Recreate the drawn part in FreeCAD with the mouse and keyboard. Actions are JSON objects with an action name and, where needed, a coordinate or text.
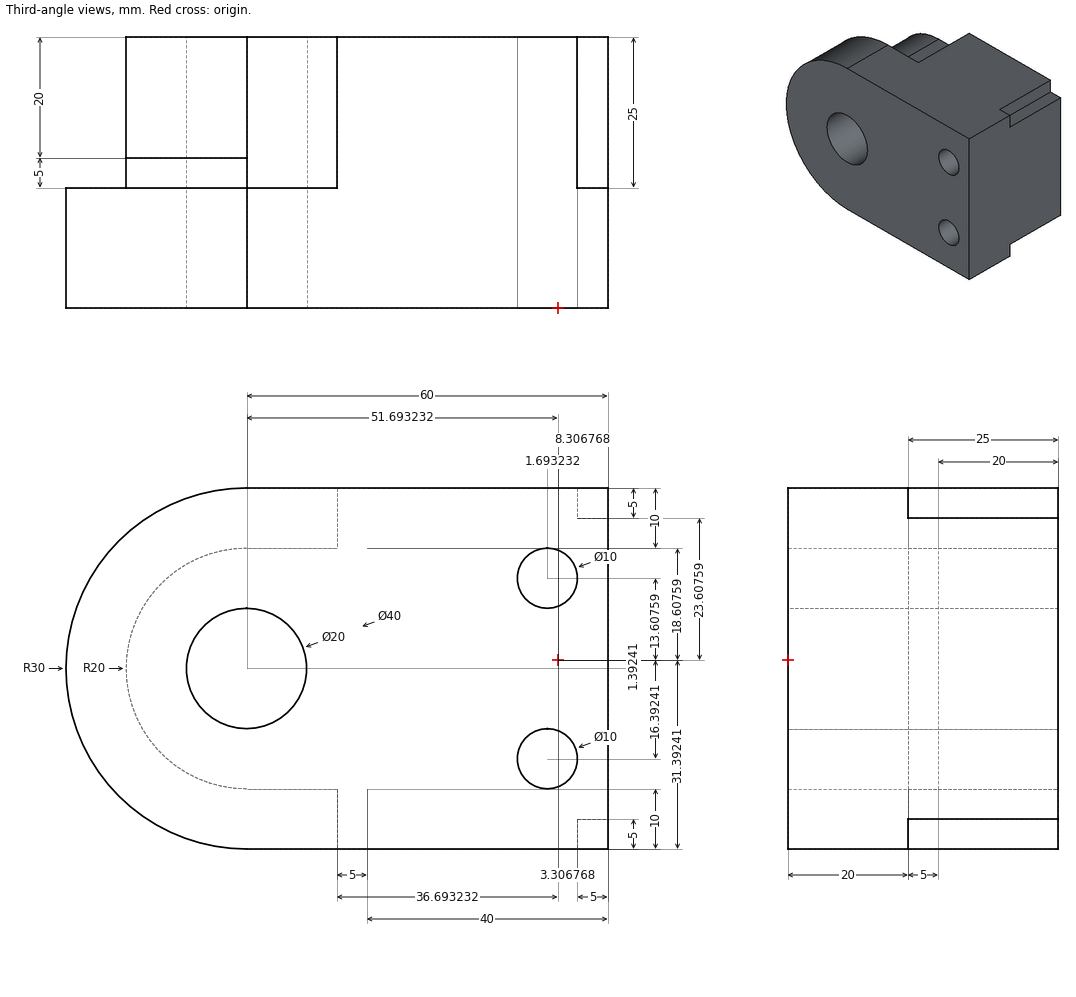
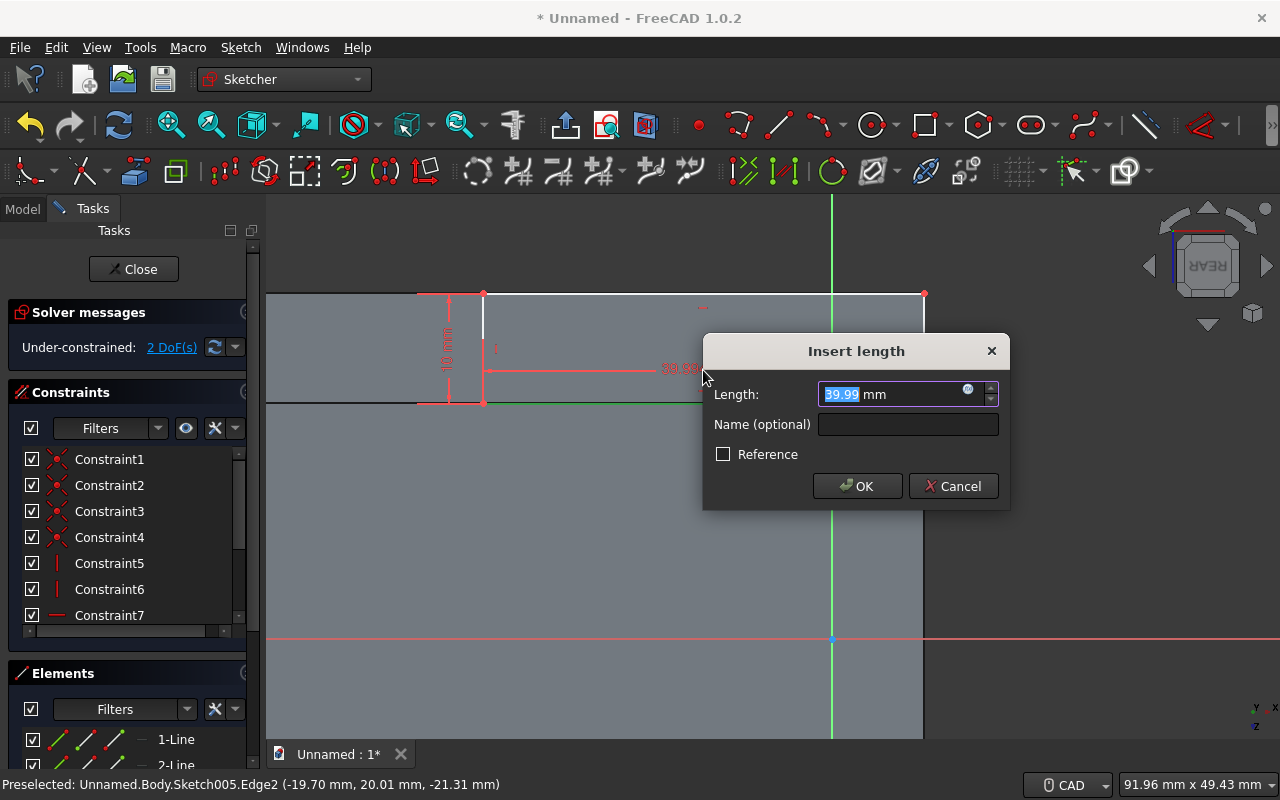
{"action": "type", "text": "40"}
{"action": "key", "text": "Return"}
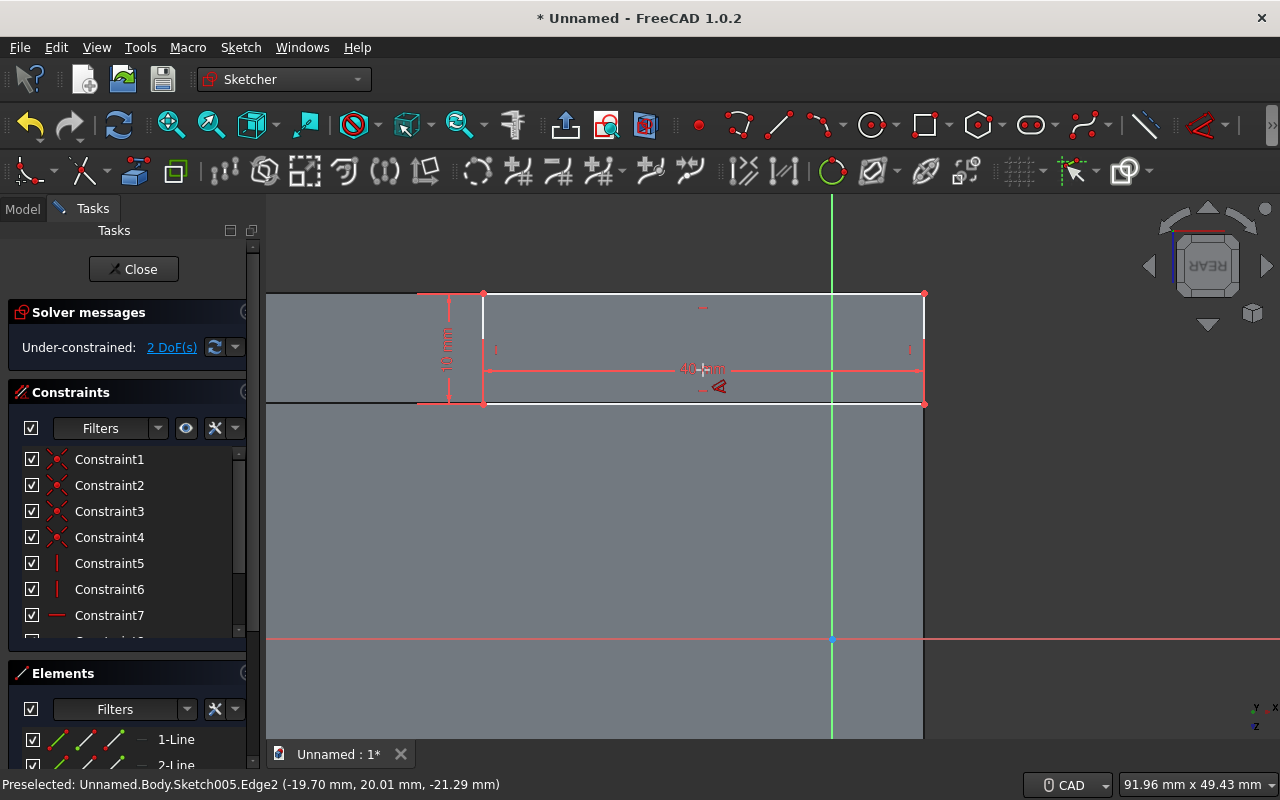
{"action": "left_click", "coordinate": [483, 294]}
{"action": "left_click", "coordinate": [449, 467]}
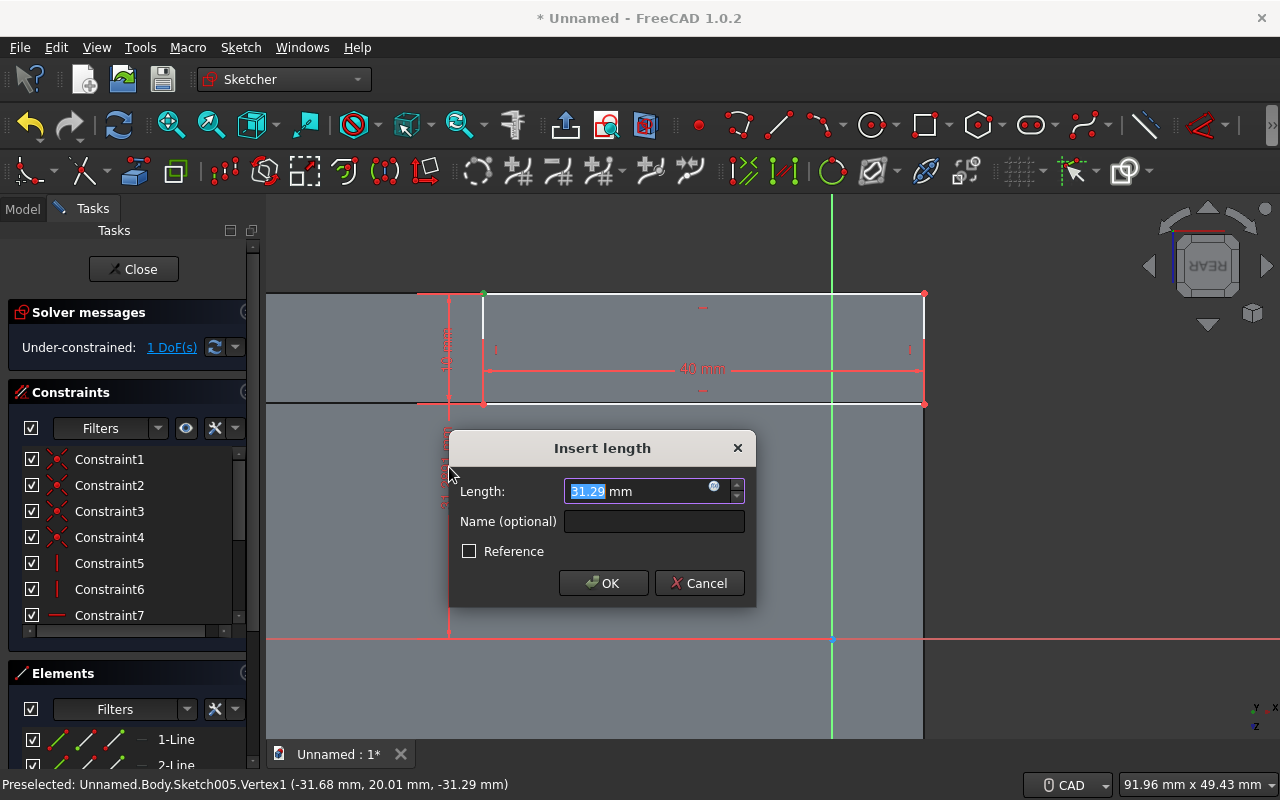
{"action": "type", "text": "31.39241"}
{"action": "key", "text": "Return"}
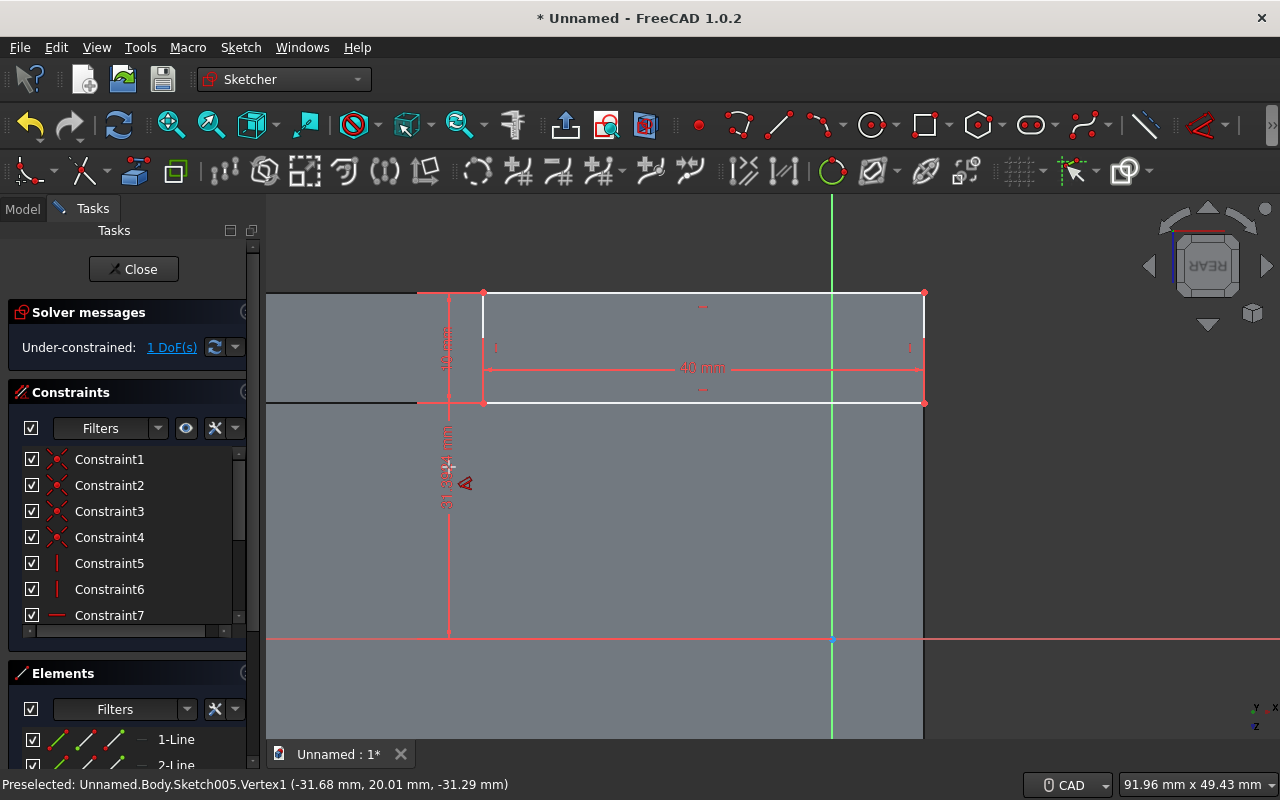
{"action": "left_click", "coordinate": [924, 403]}
{"action": "left_click", "coordinate": [878, 673]}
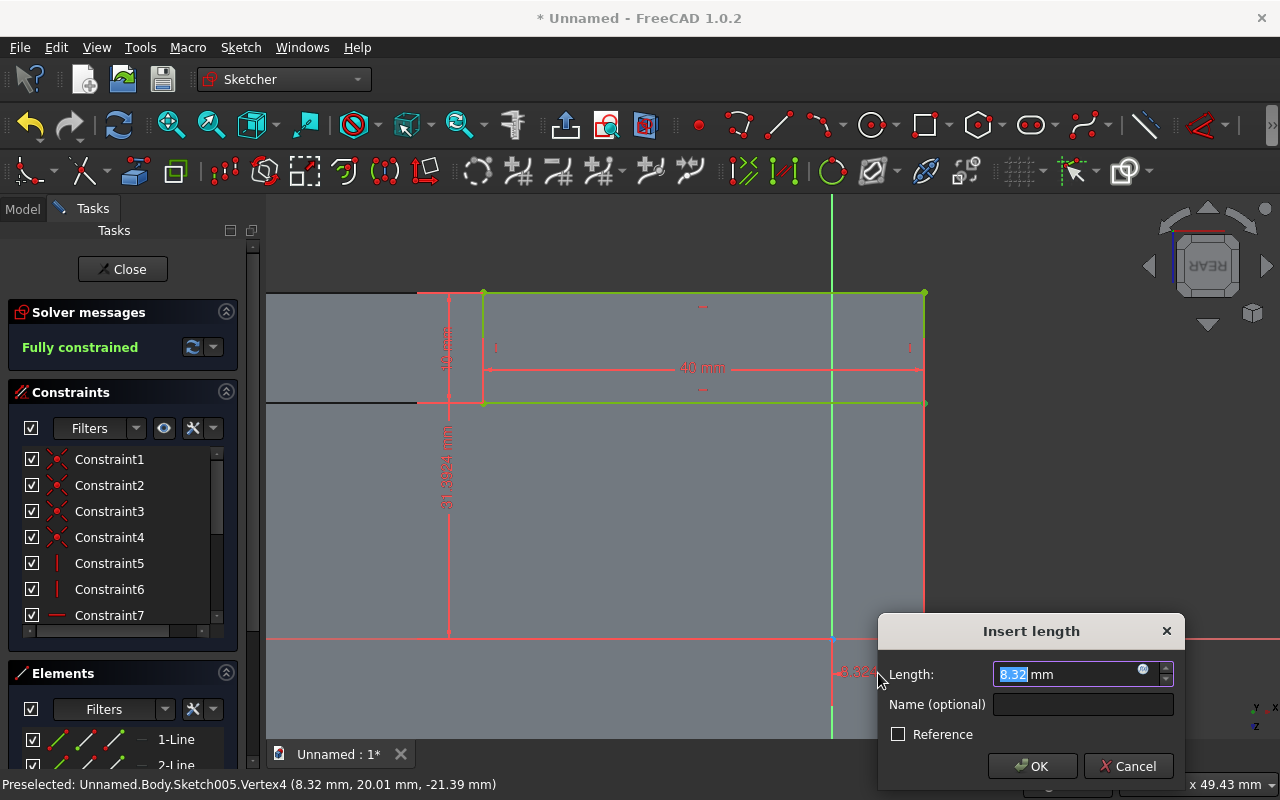
{"action": "type", "text": "8.306768"}
{"action": "key", "text": "Return"}
{"action": "key", "text": "Escape"}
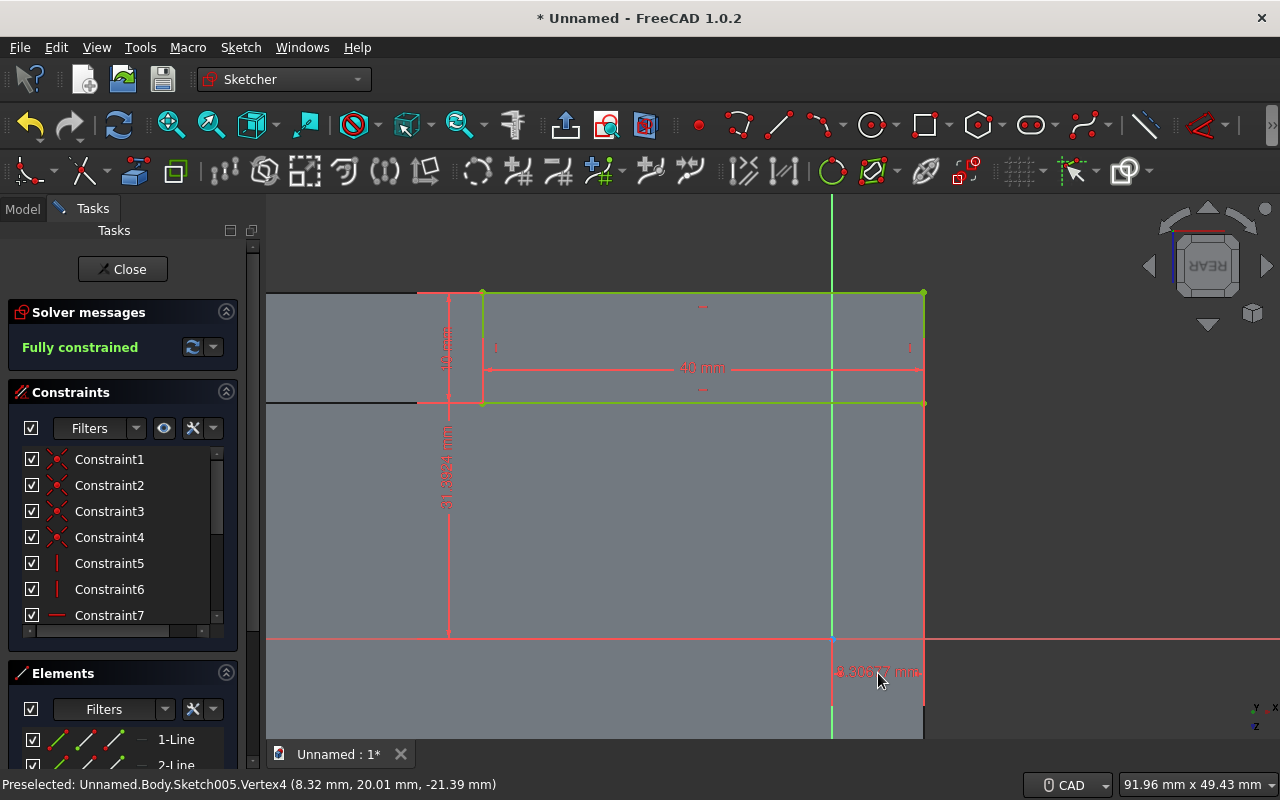
{"action": "left_click", "coordinate": [123, 269]}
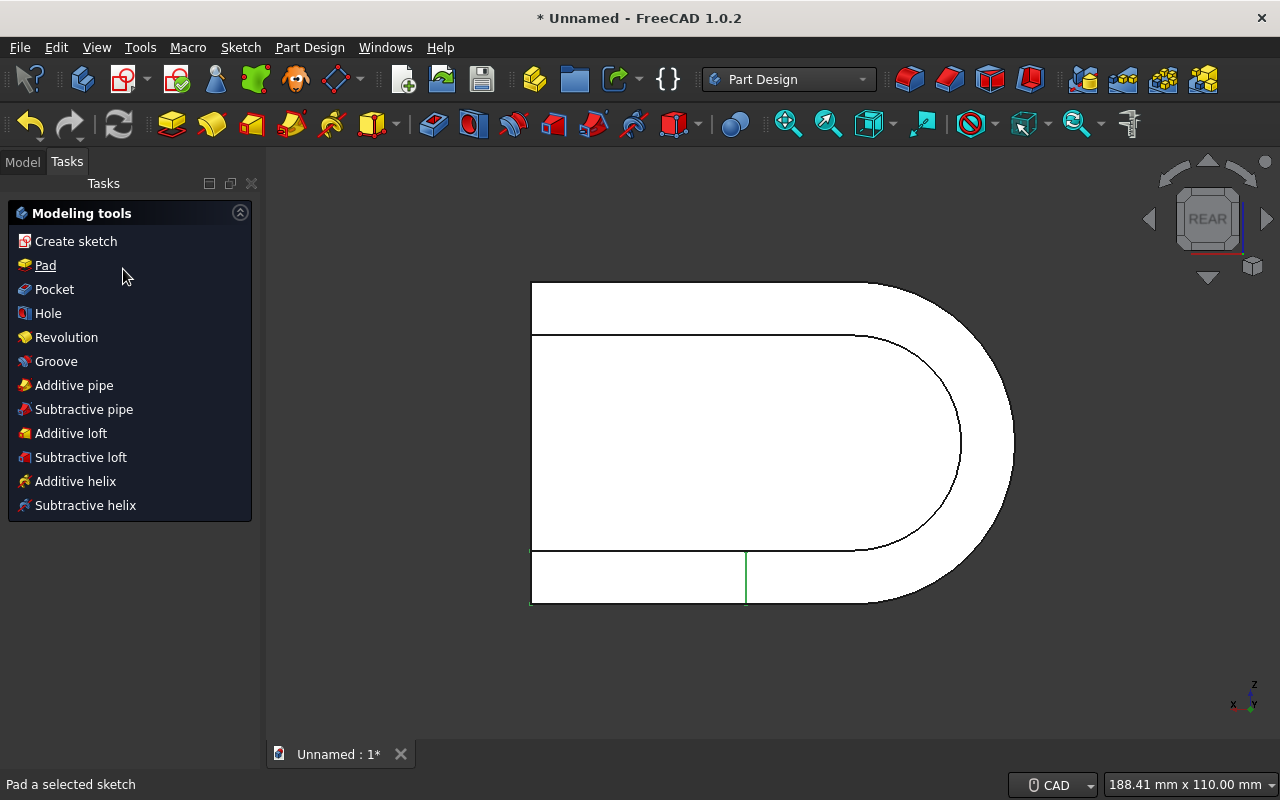
{"action": "left_click", "coordinate": [172, 124]}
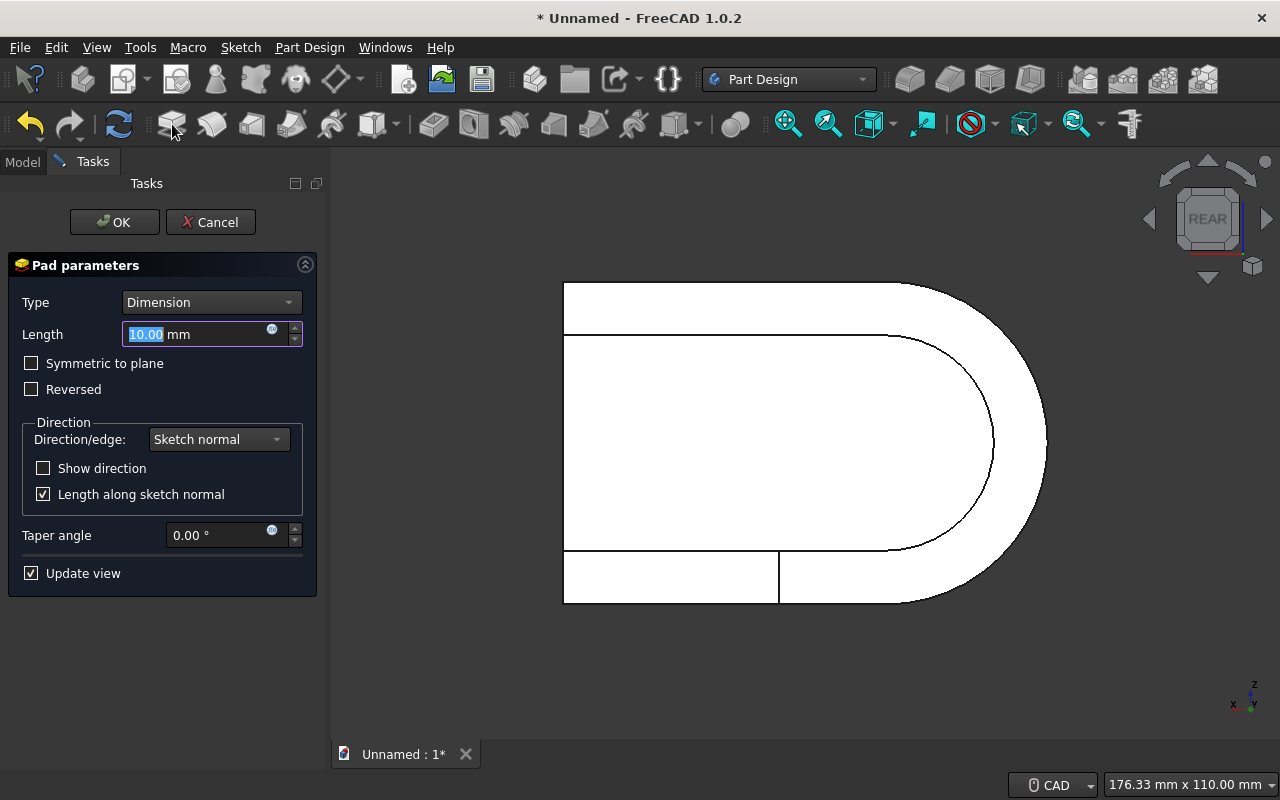
{"action": "type", "text": "5"}
{"action": "key", "text": "Tab"}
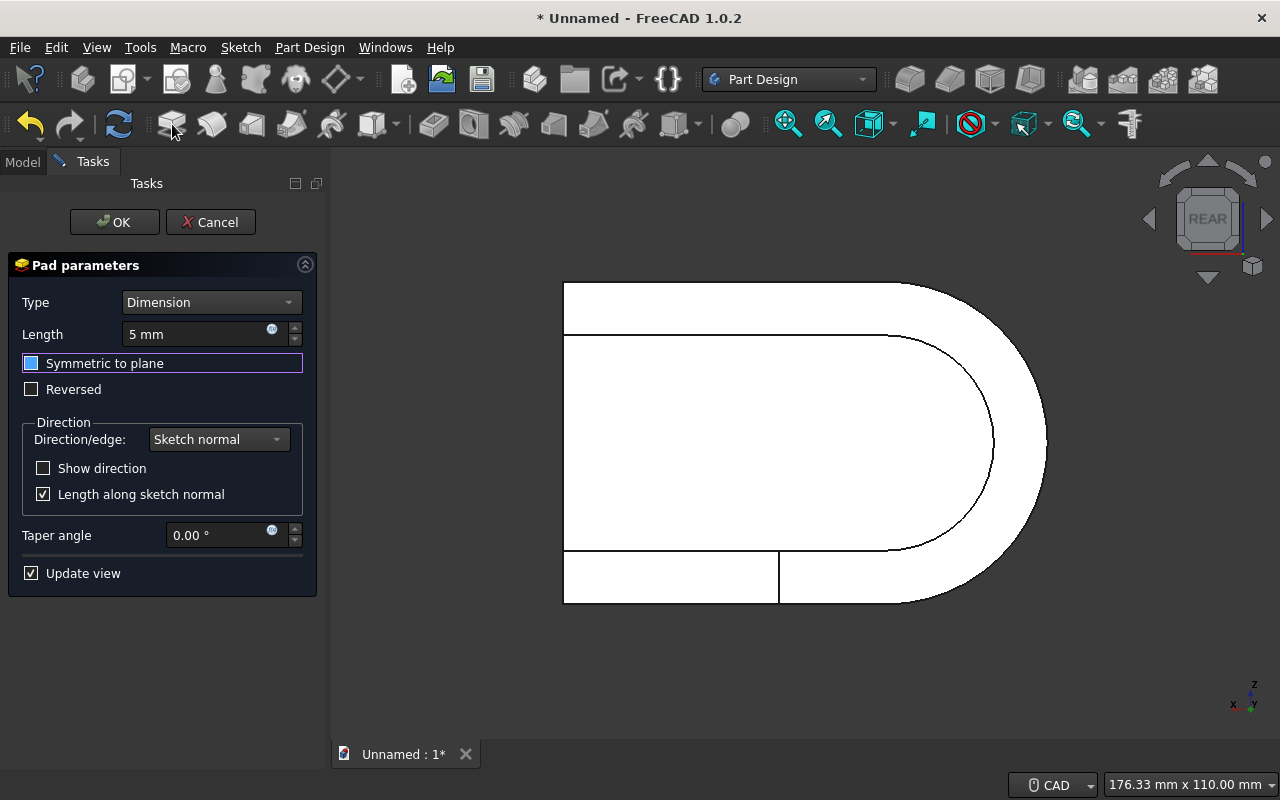
{"action": "left_click", "coordinate": [115, 222]}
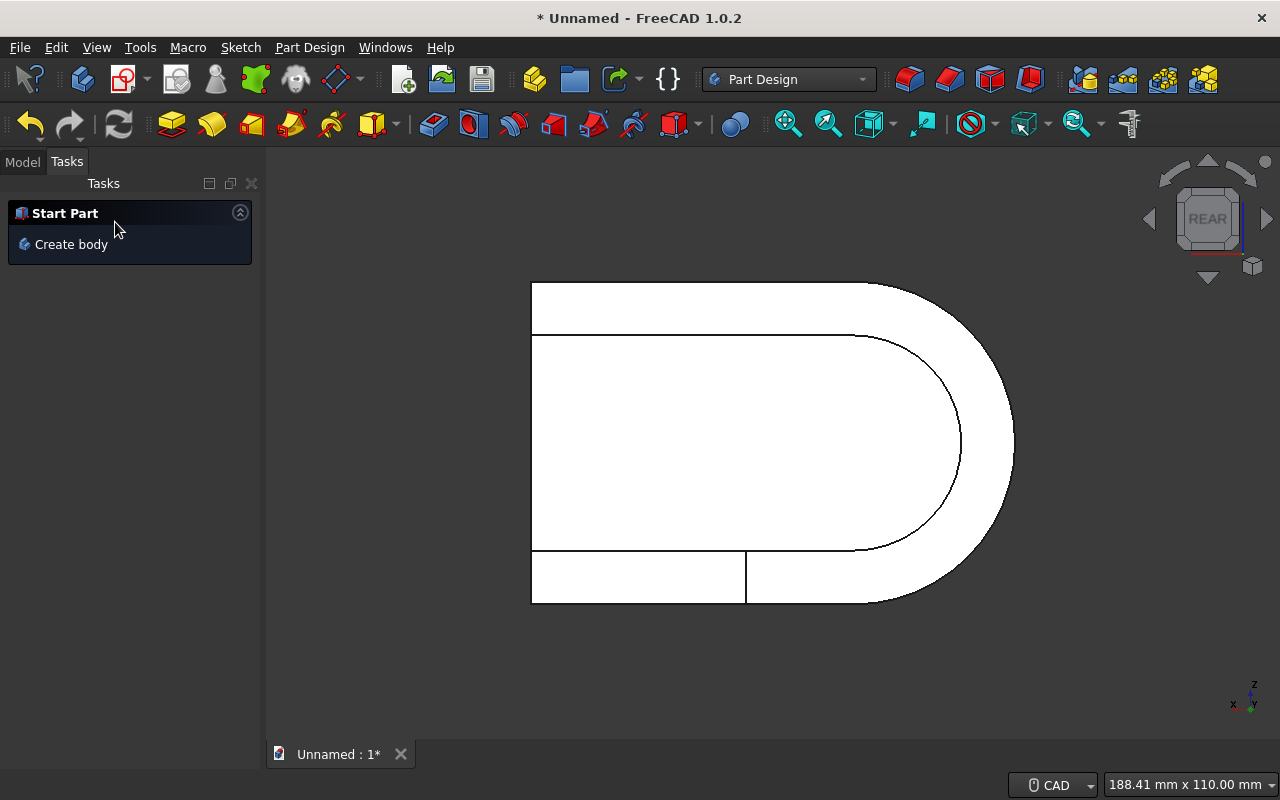
{"action": "left_click", "coordinate": [577, 577]}